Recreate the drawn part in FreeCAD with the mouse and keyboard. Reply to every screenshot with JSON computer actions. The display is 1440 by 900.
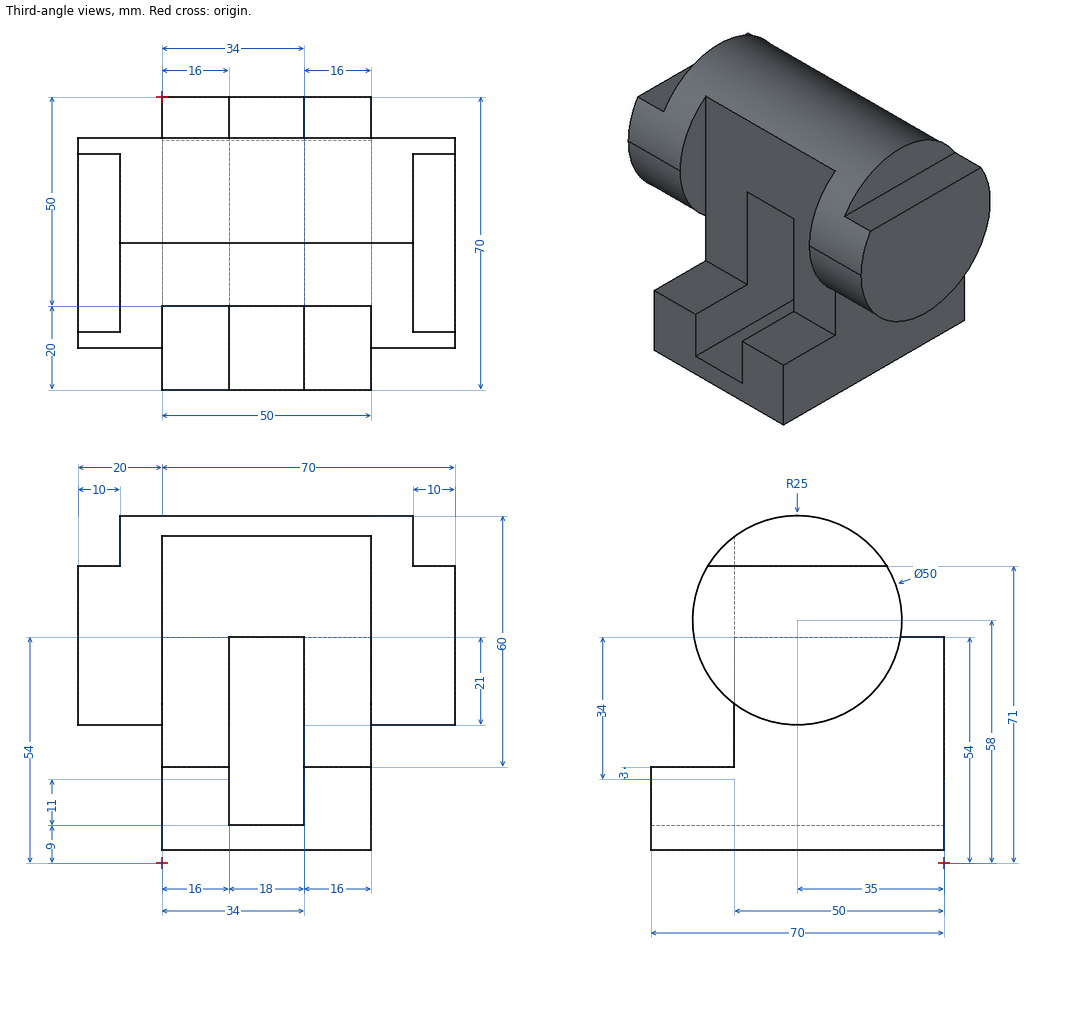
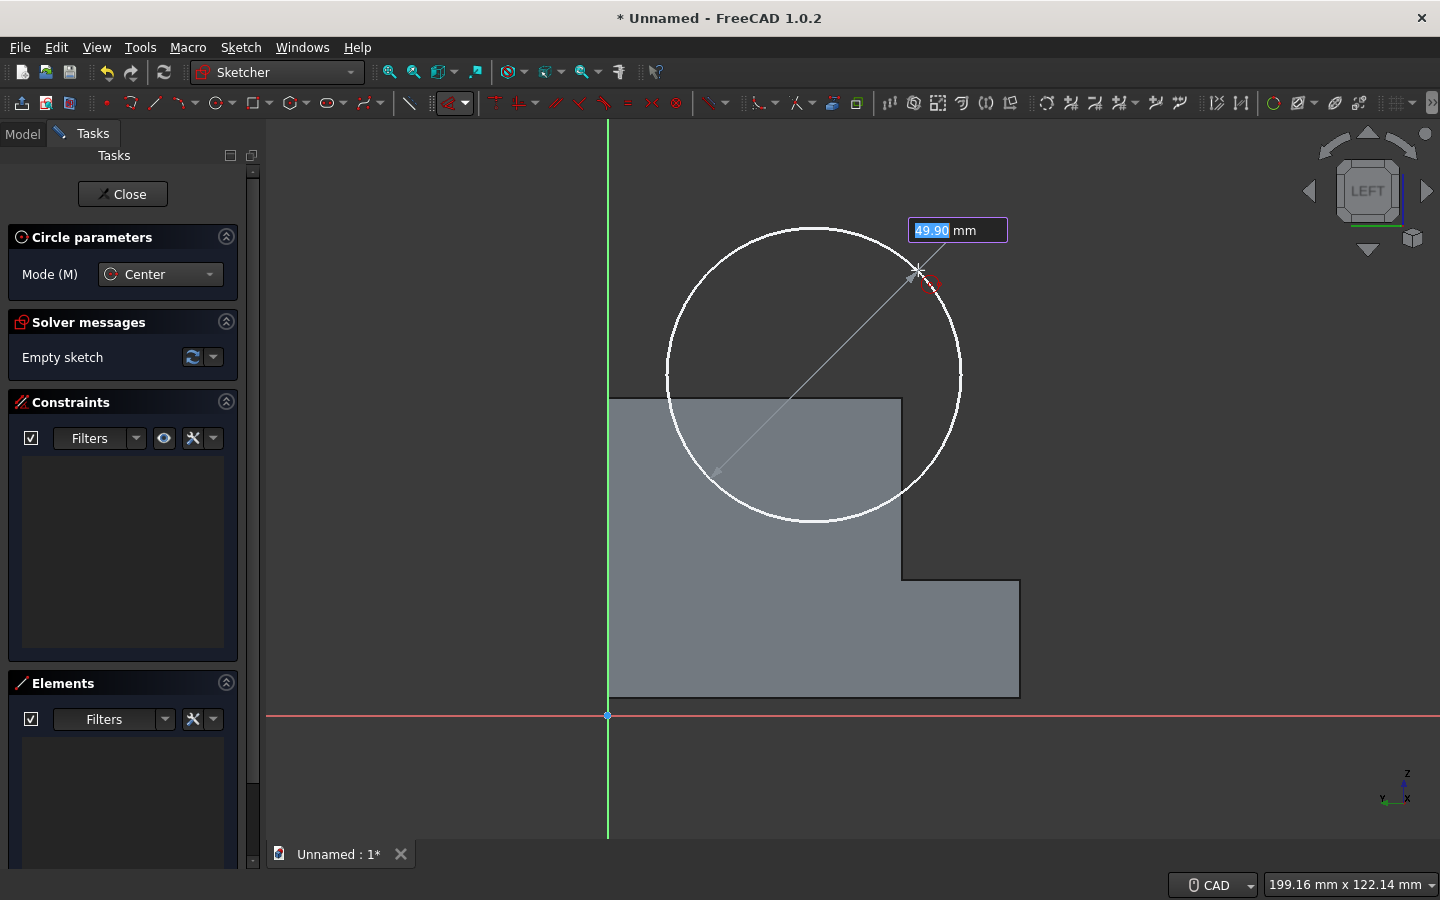
{"action": "type", "text": "50"}
{"action": "key", "text": "Return"}
{"action": "key", "text": "Escape"}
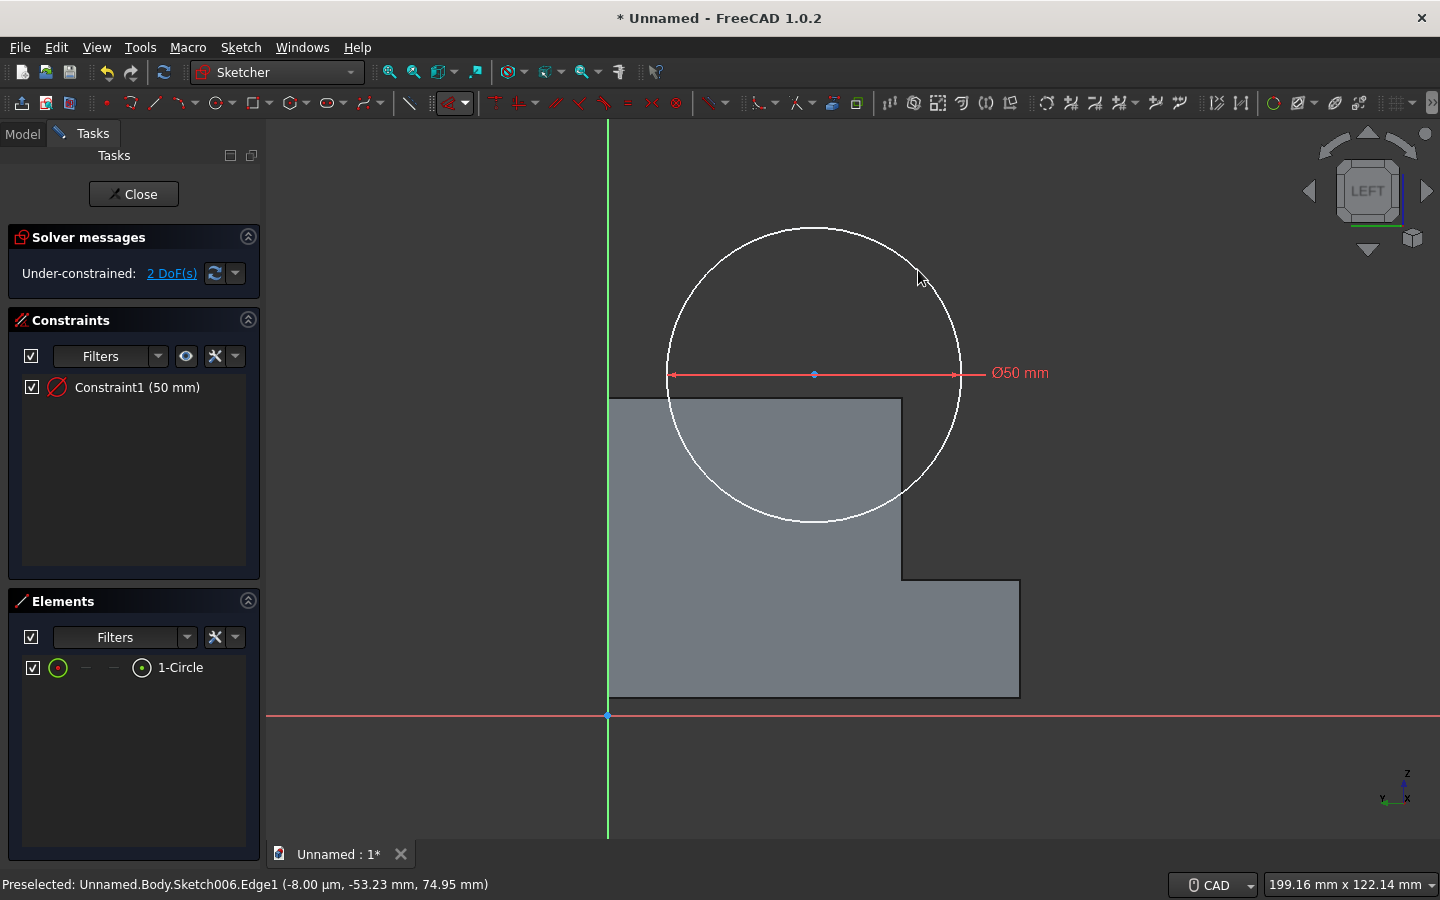
{"action": "left_click", "coordinate": [814, 375]}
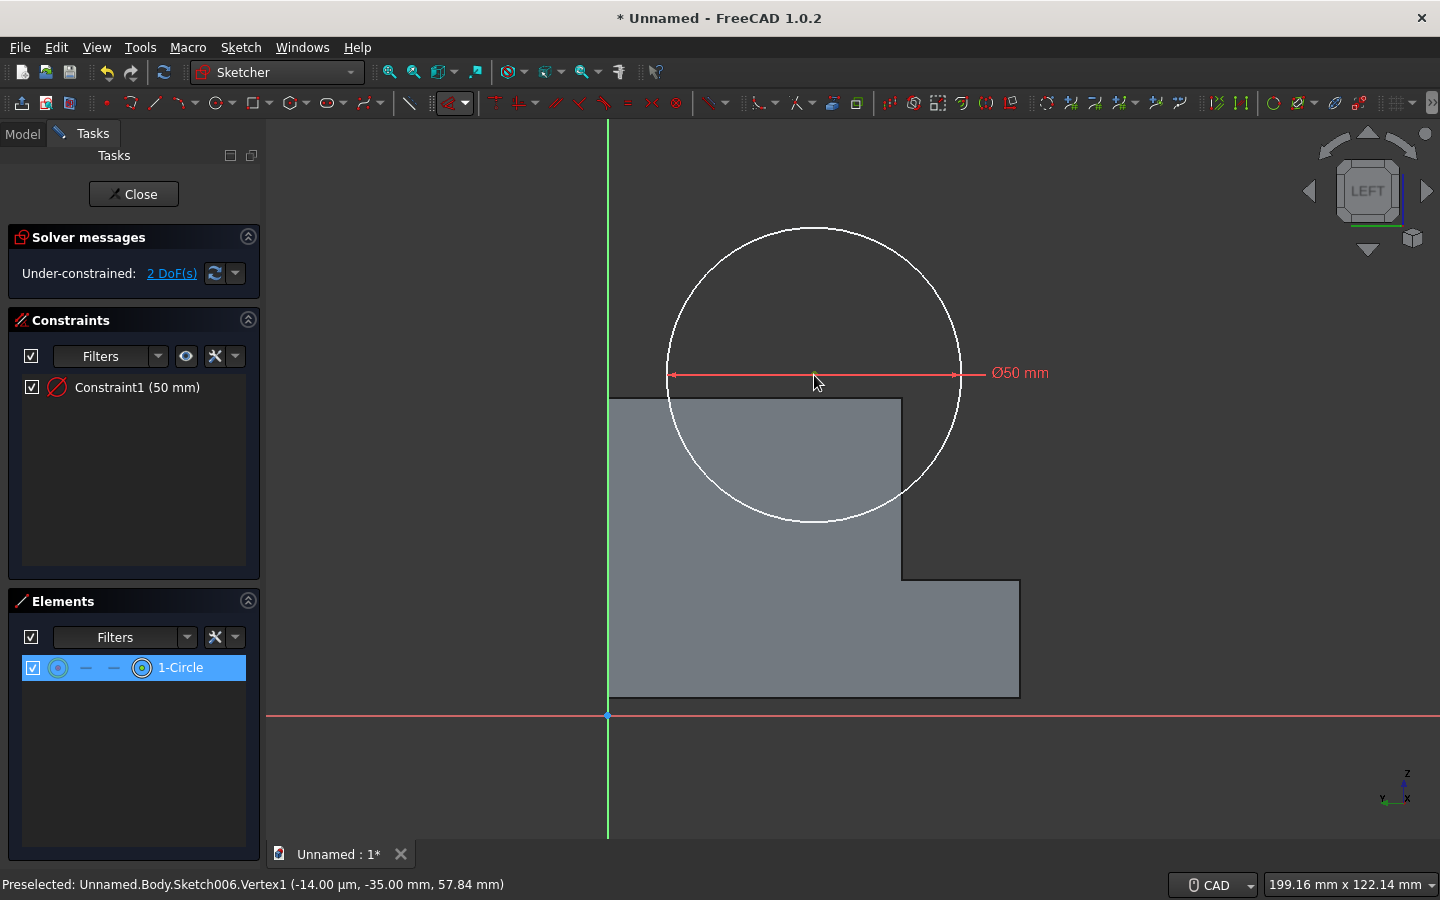
{"action": "key", "text": "l"}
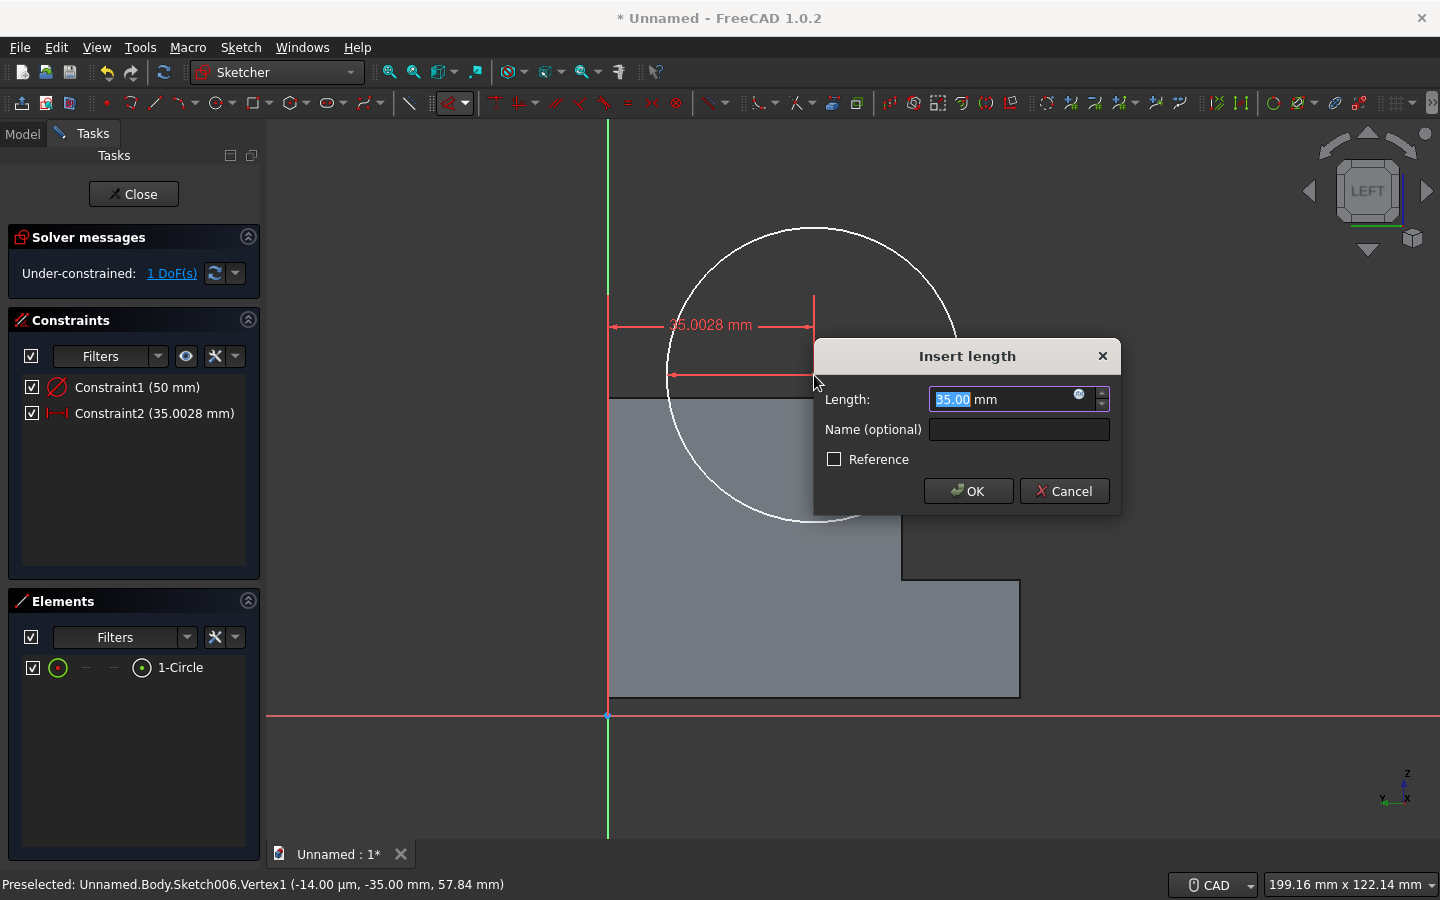
{"action": "type", "text": "35"}
{"action": "key", "text": "Return"}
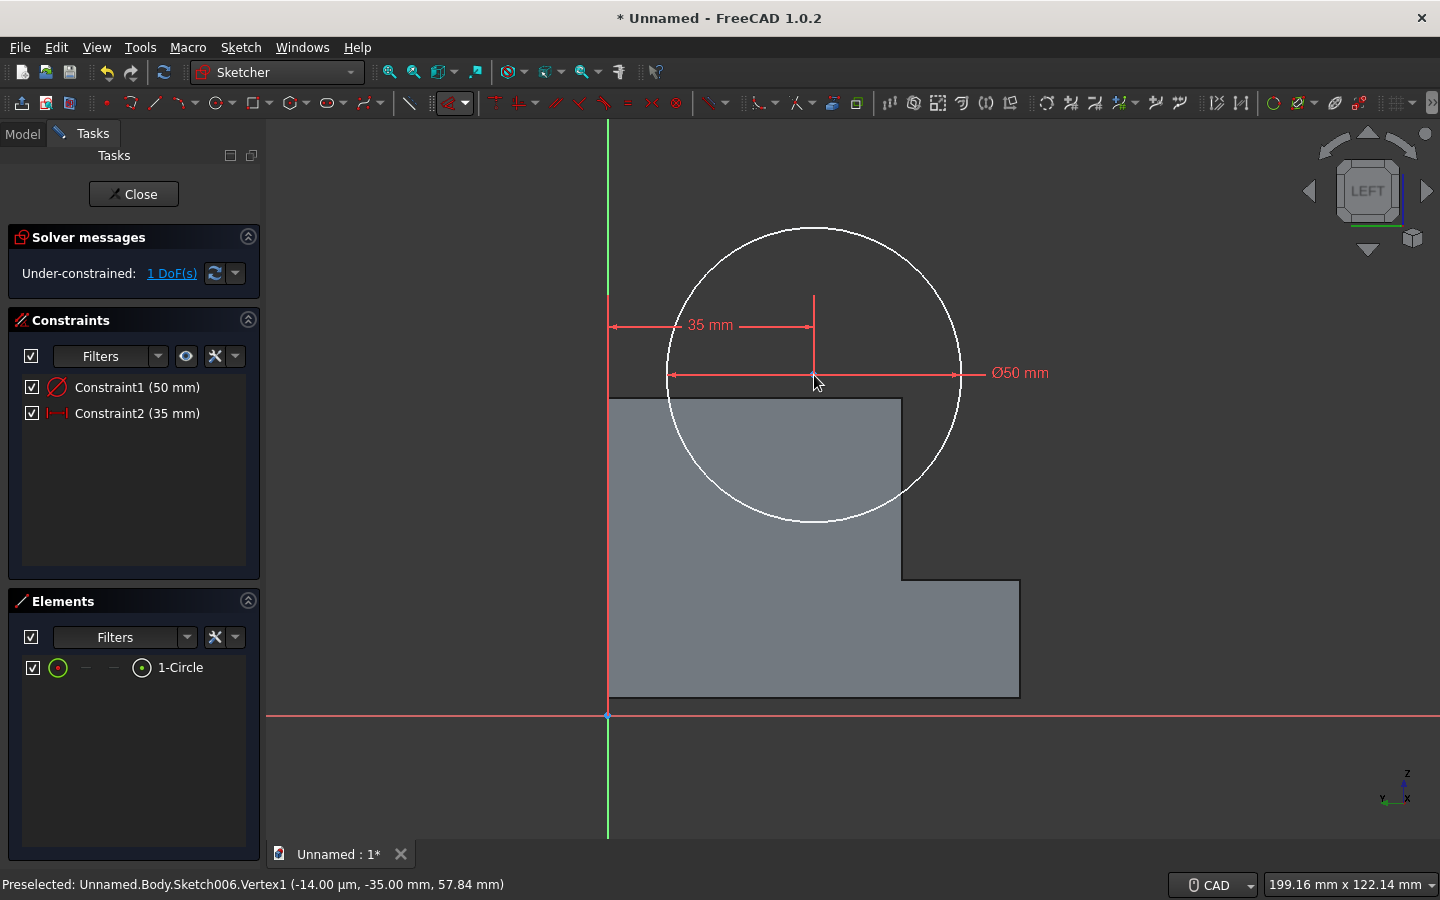
{"action": "left_click", "coordinate": [814, 375]}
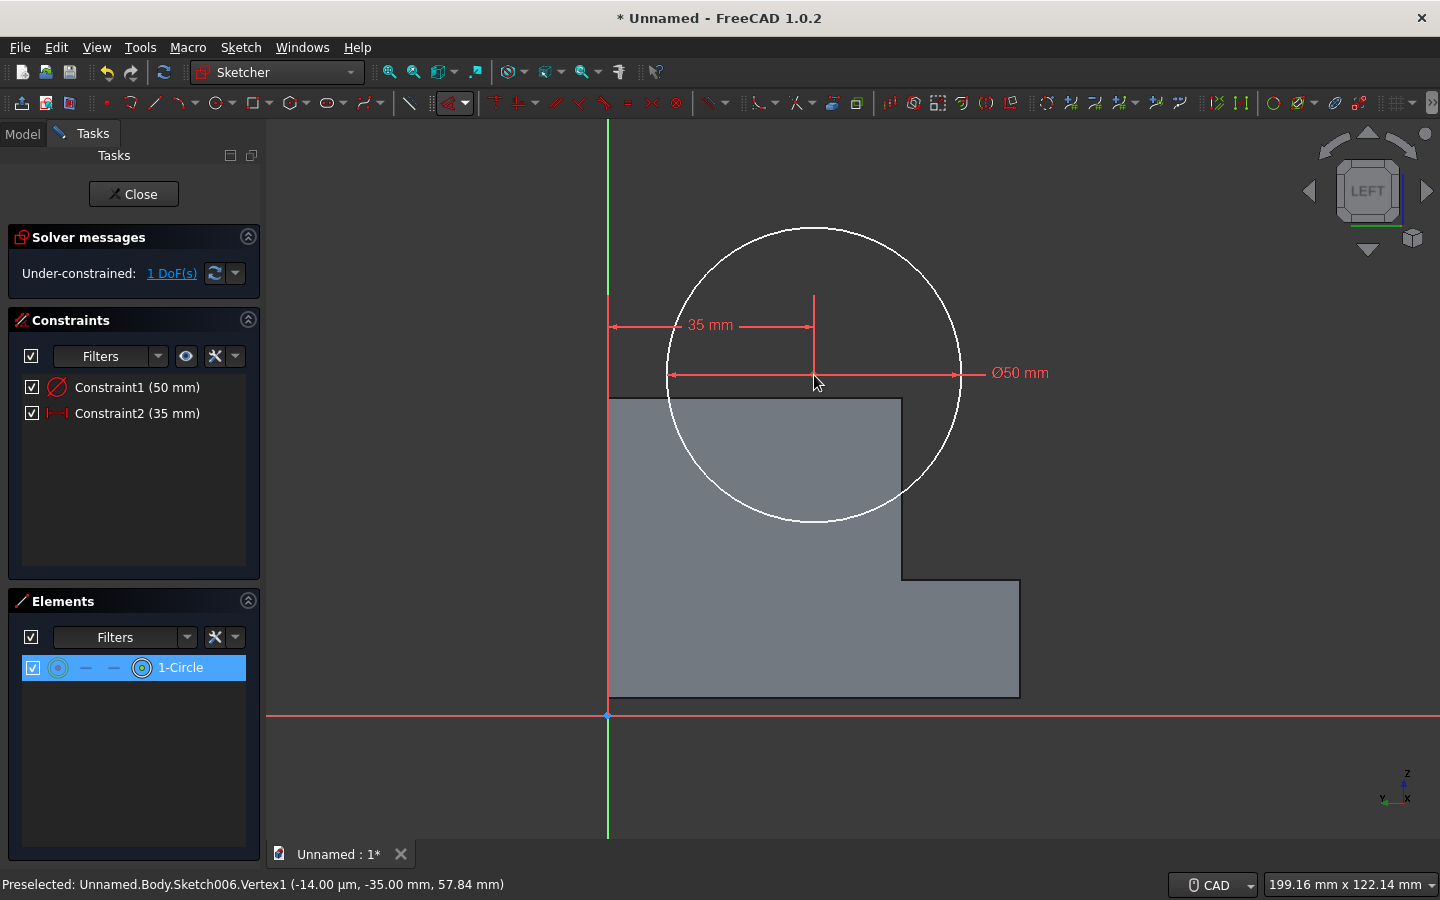
{"action": "key", "text": "i"}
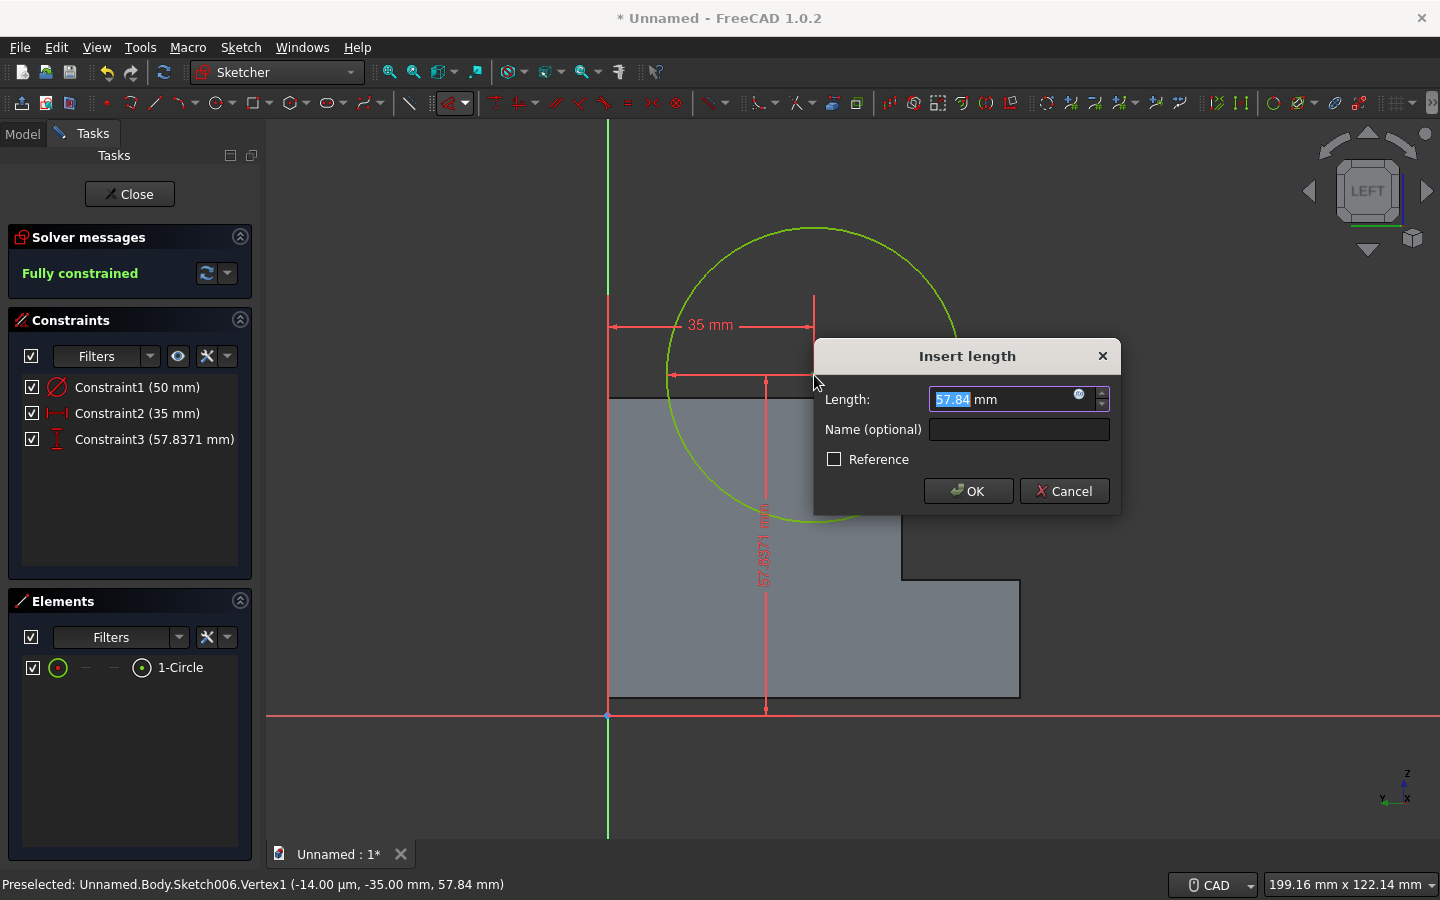
{"action": "type", "text": "58"}
{"action": "key", "text": "Return"}